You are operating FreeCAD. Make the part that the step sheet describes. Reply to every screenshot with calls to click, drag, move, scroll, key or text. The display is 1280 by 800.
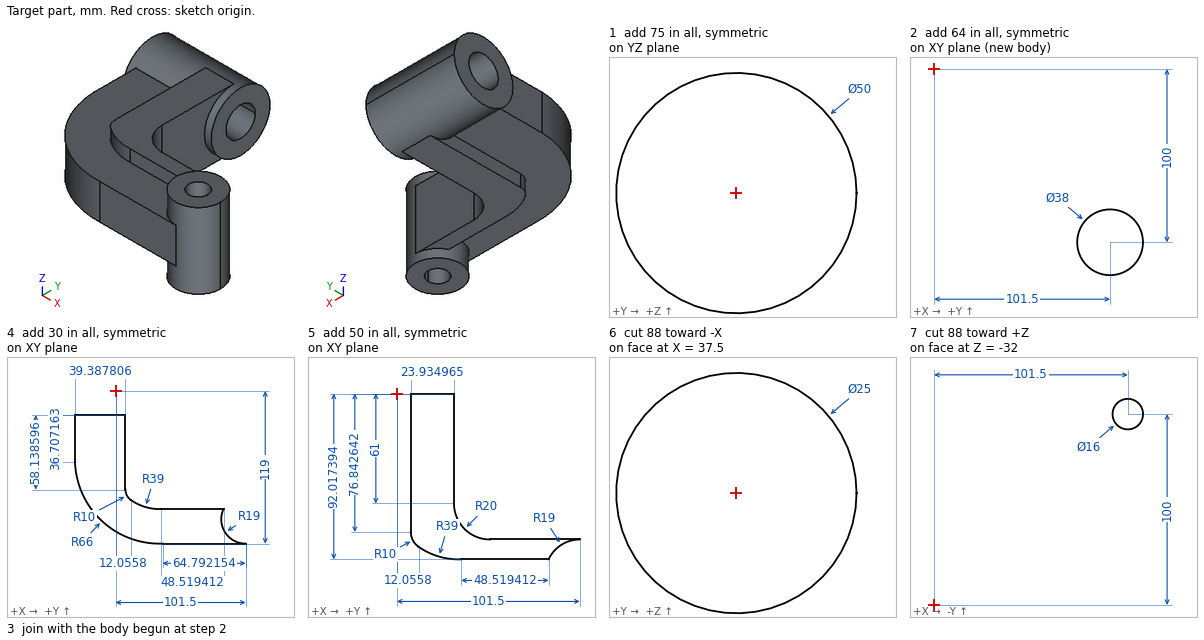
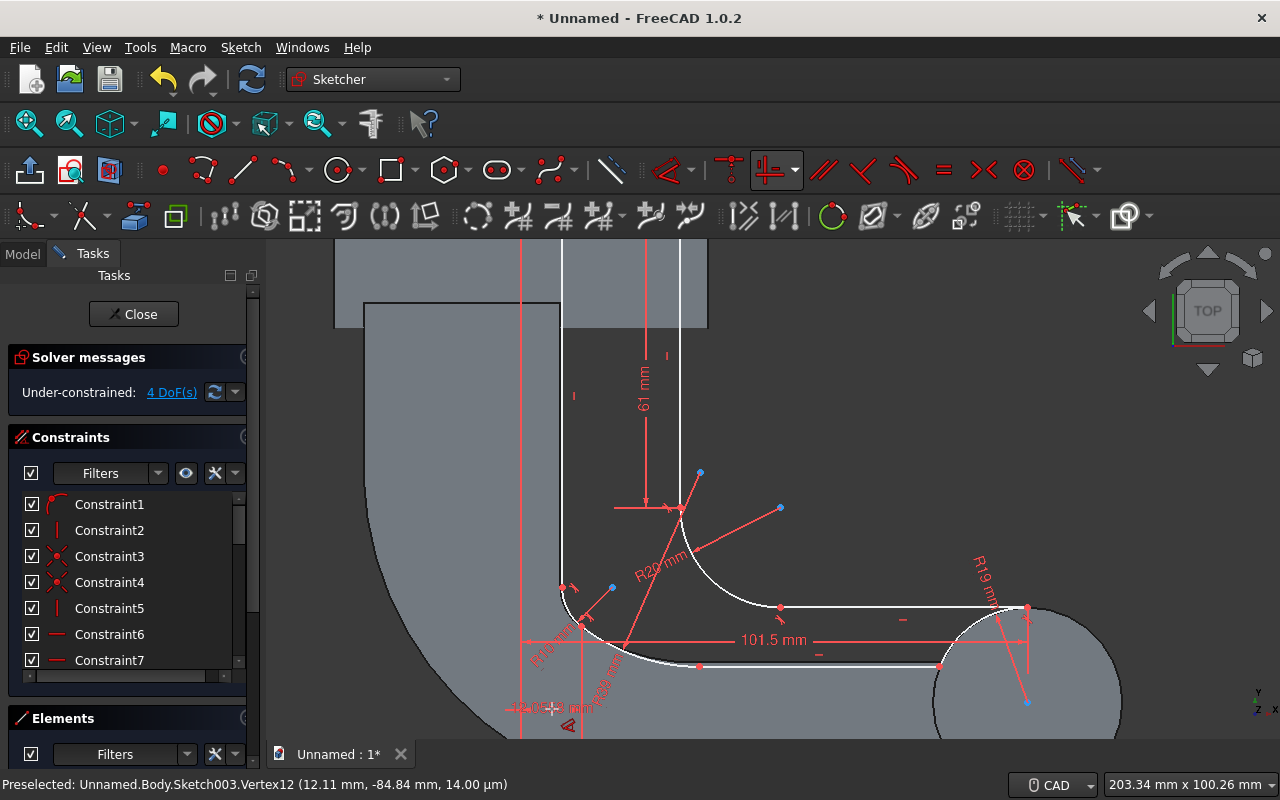
scroll(562, 603, down, 2)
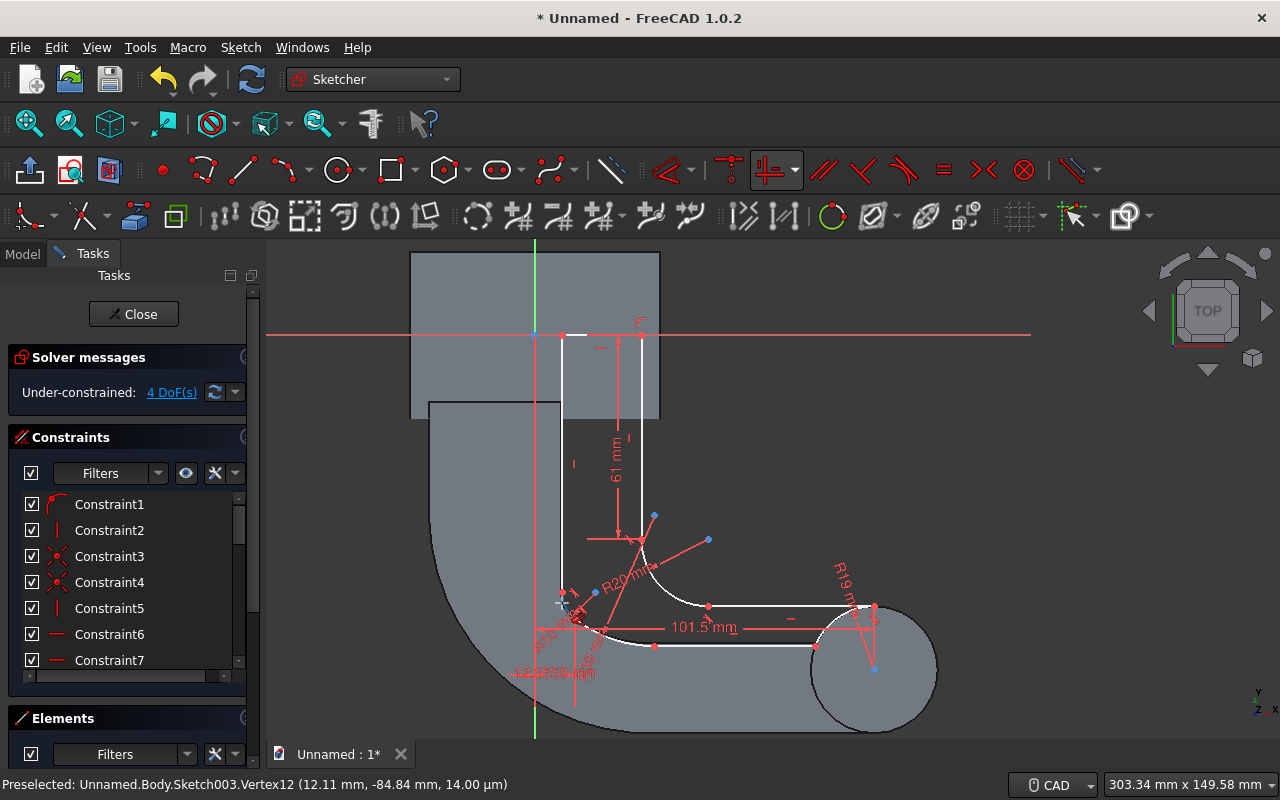
click(618, 335)
click(602, 301)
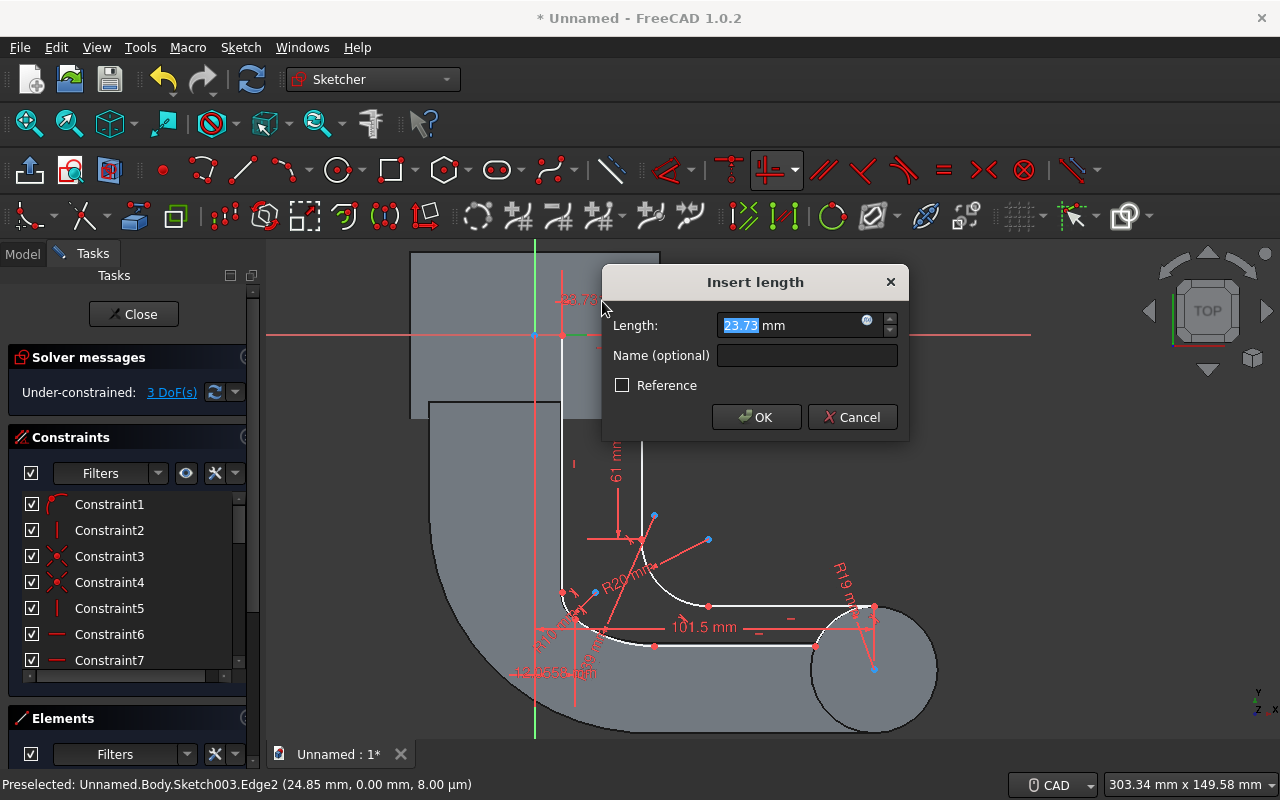
text(23.934965)
key(Return)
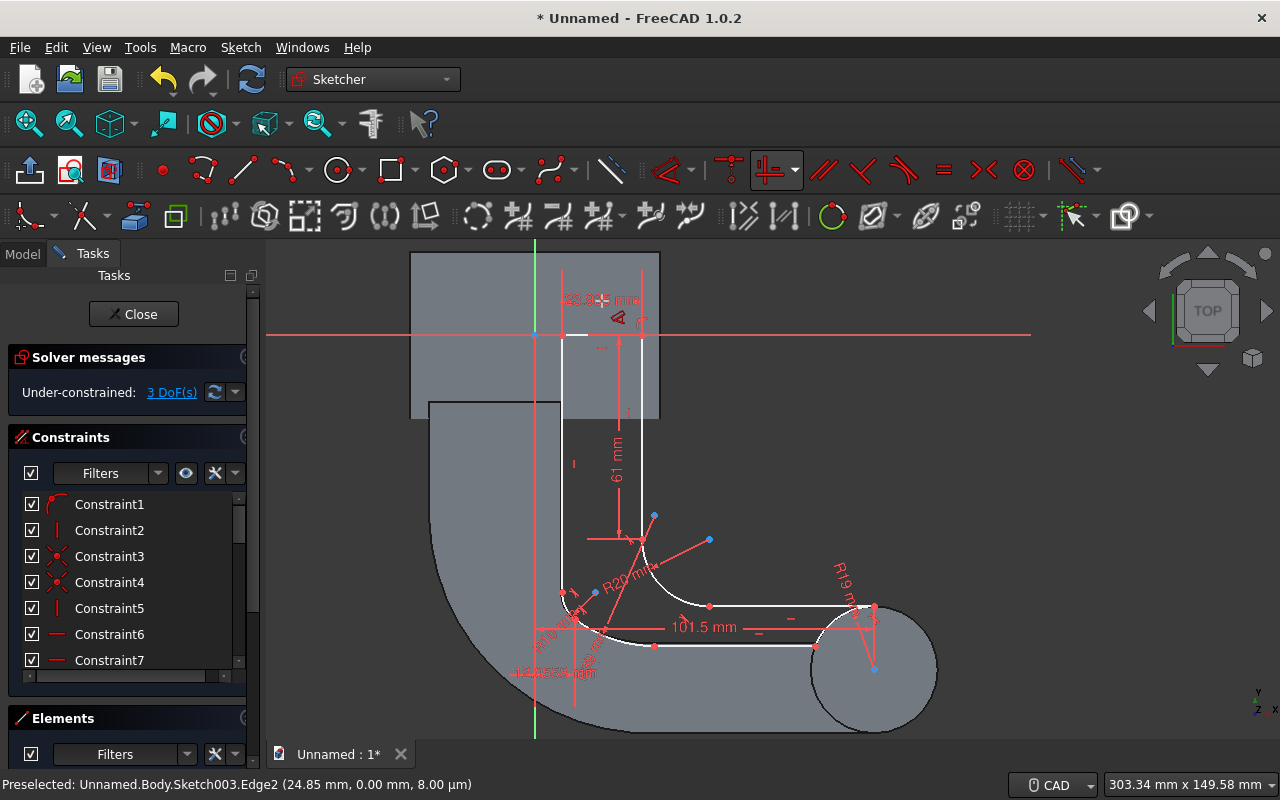
click(562, 413)
click(596, 405)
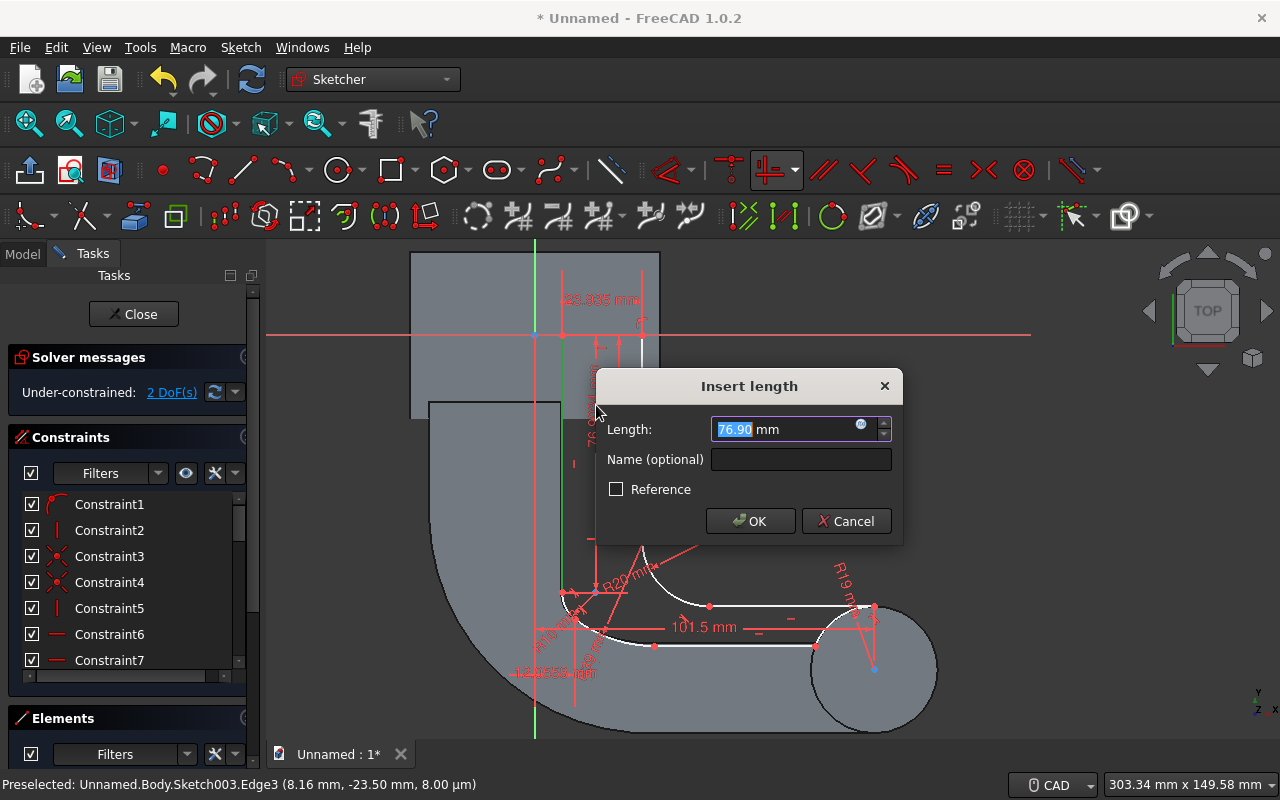
text(76.842642)
key(Return)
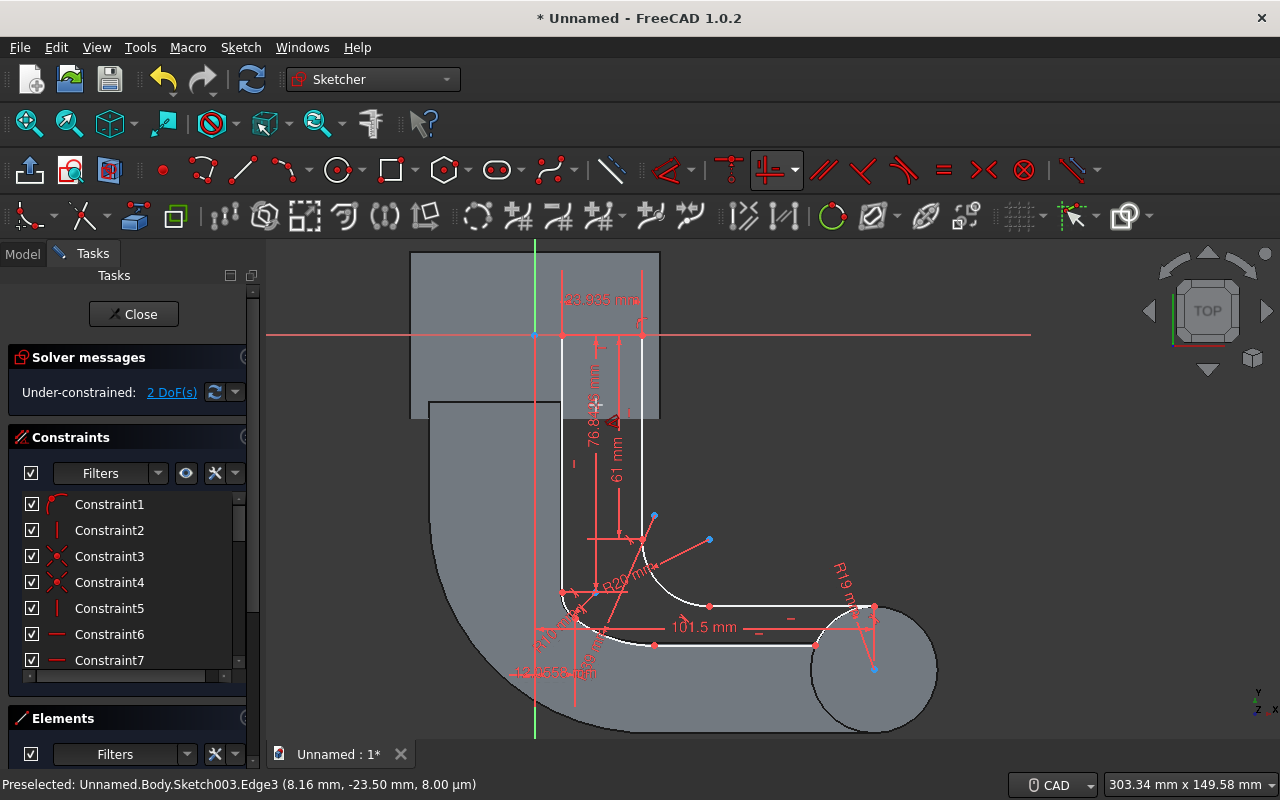
click(703, 646)
click(735, 680)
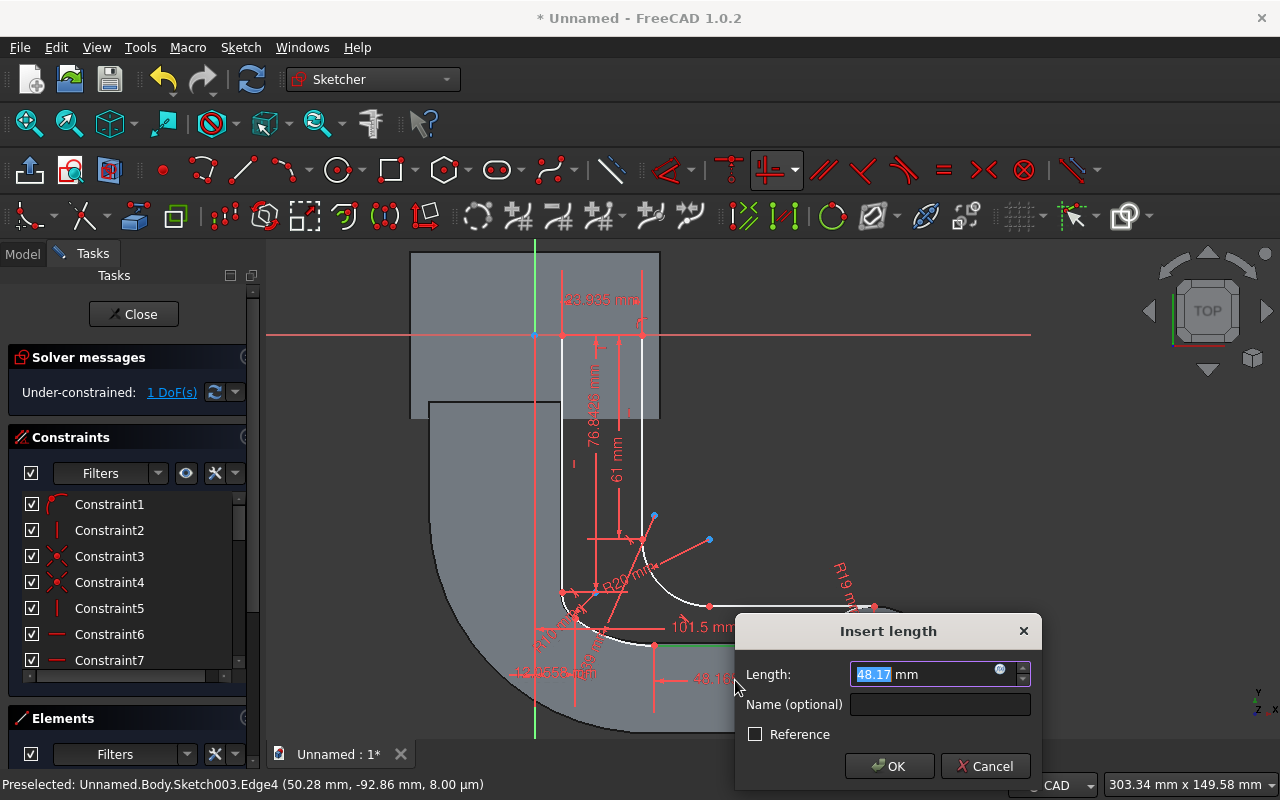
text(48.519412)
key(Return)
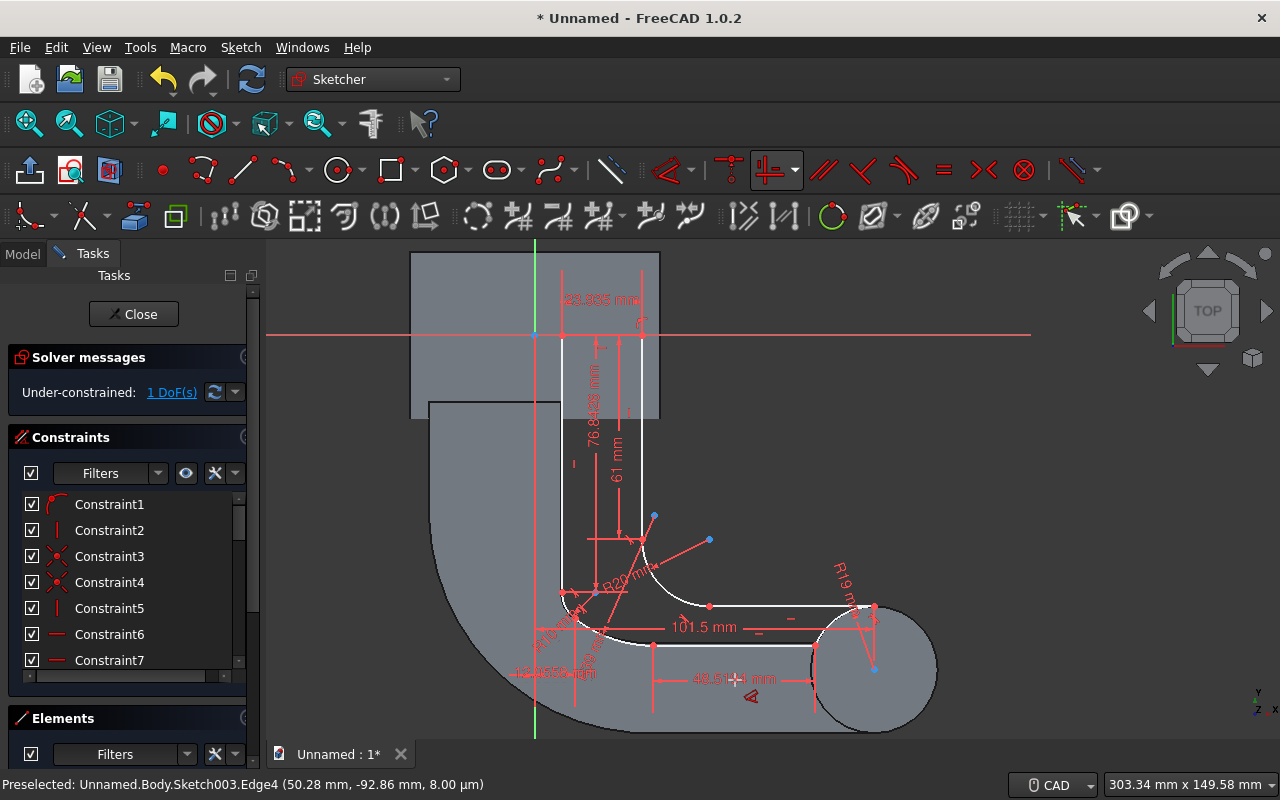
click(653, 646)
click(501, 491)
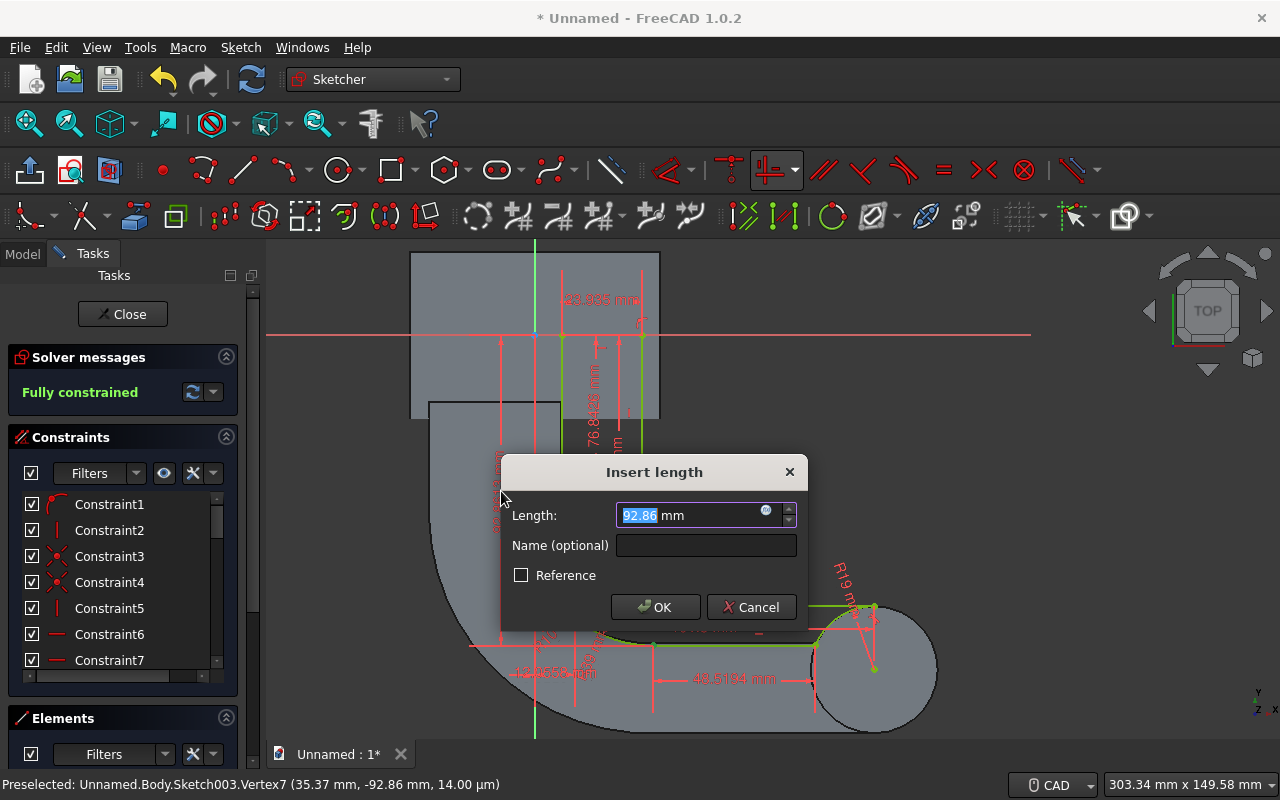
text(92.017394)
key(Return)
key(Escape)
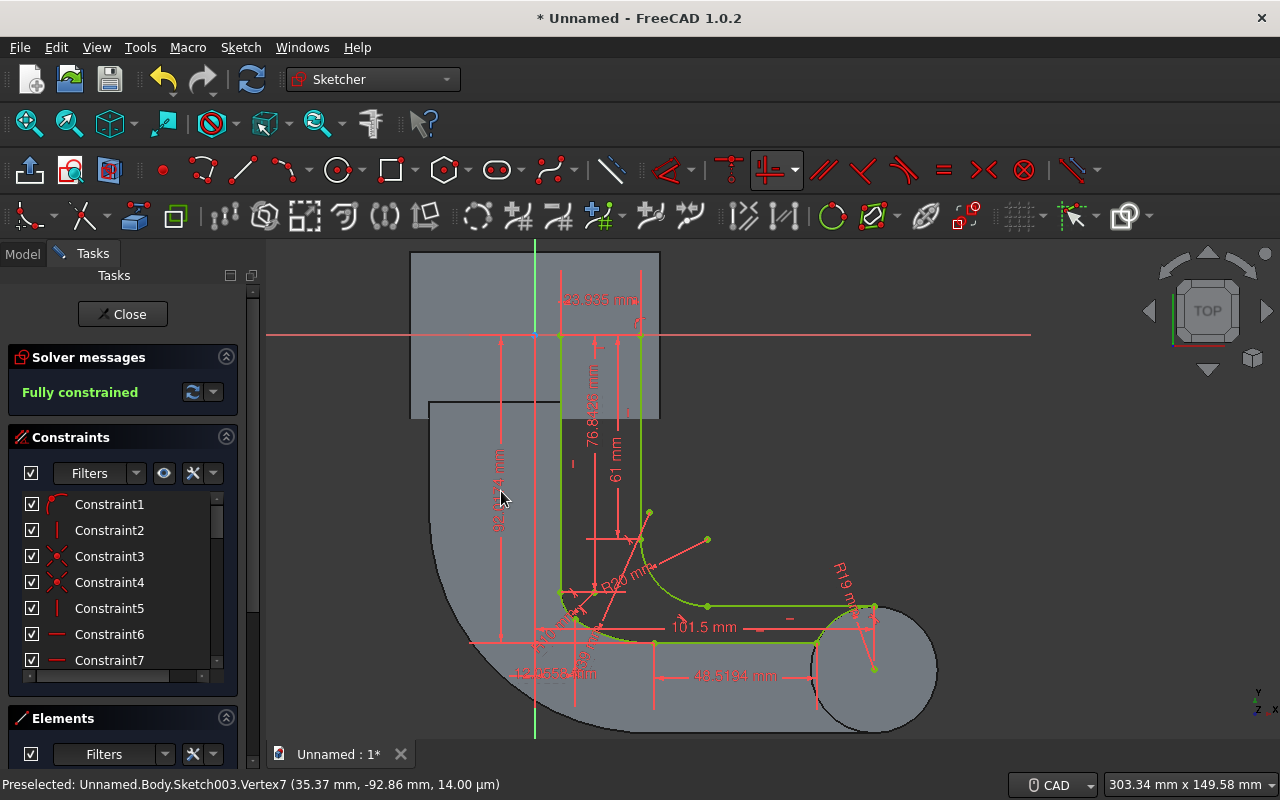
click(123, 314)